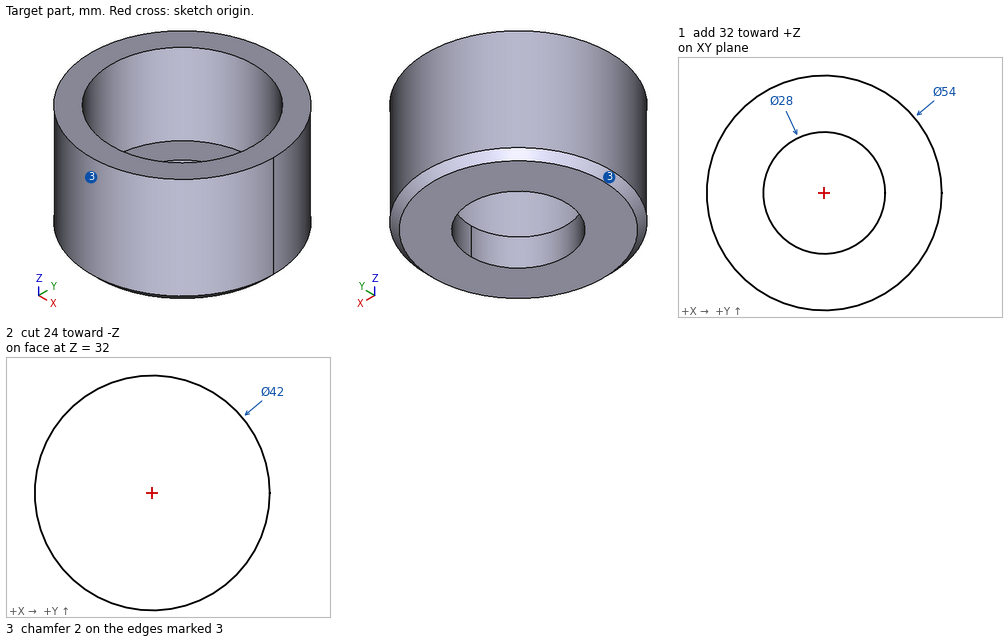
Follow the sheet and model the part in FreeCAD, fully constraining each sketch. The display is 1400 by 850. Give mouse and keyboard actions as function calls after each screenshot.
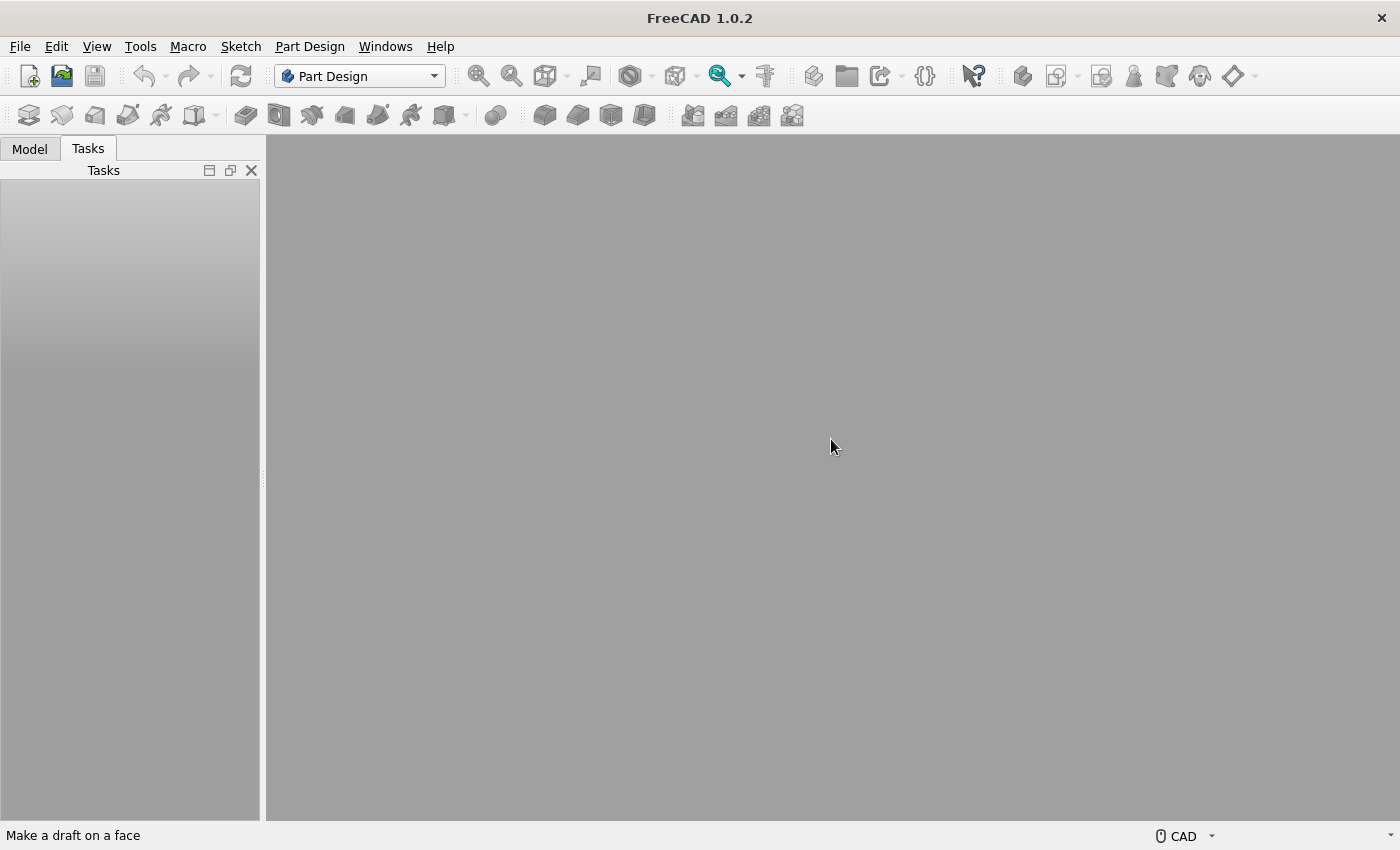
key(ctrl+n)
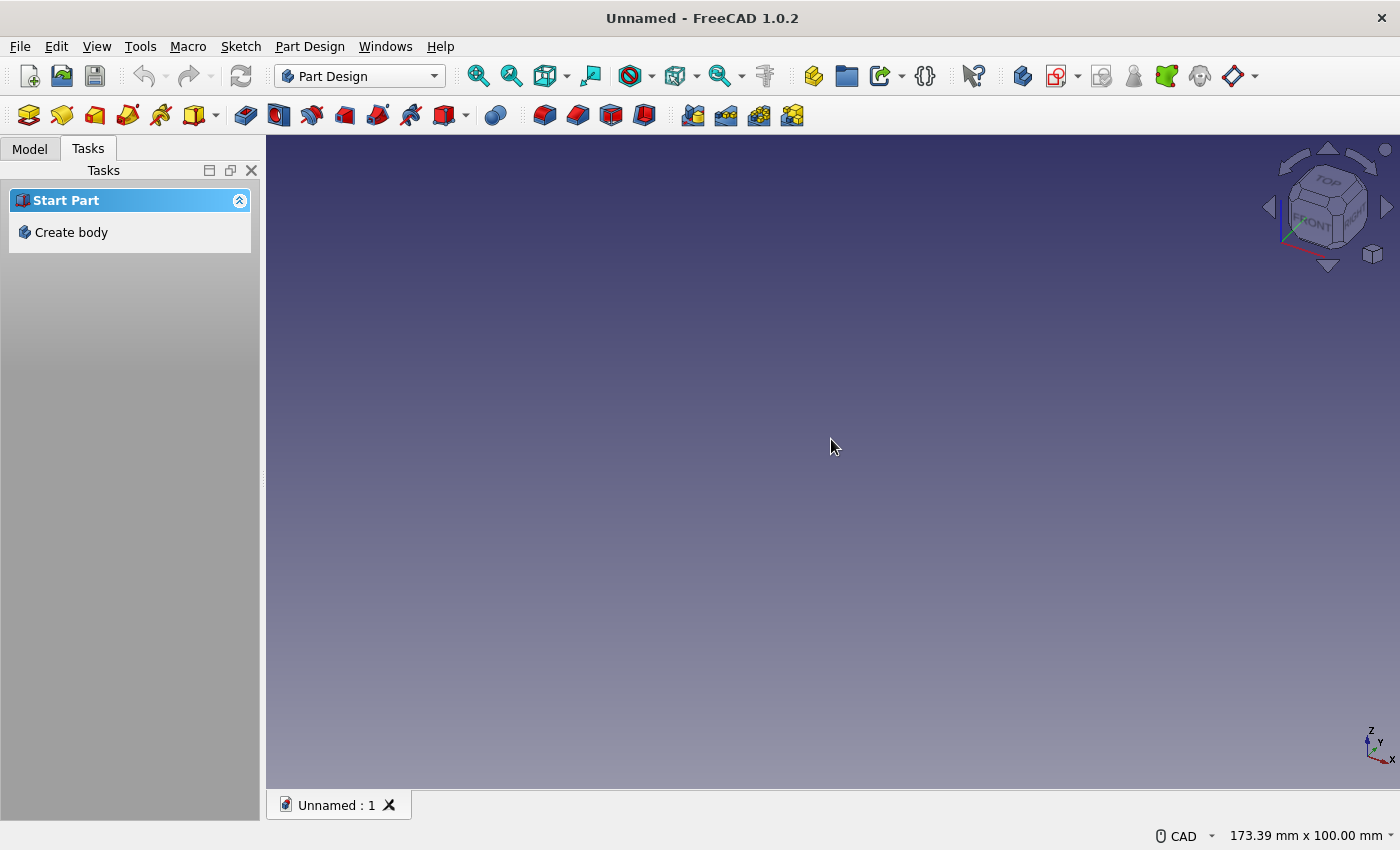
click(1056, 76)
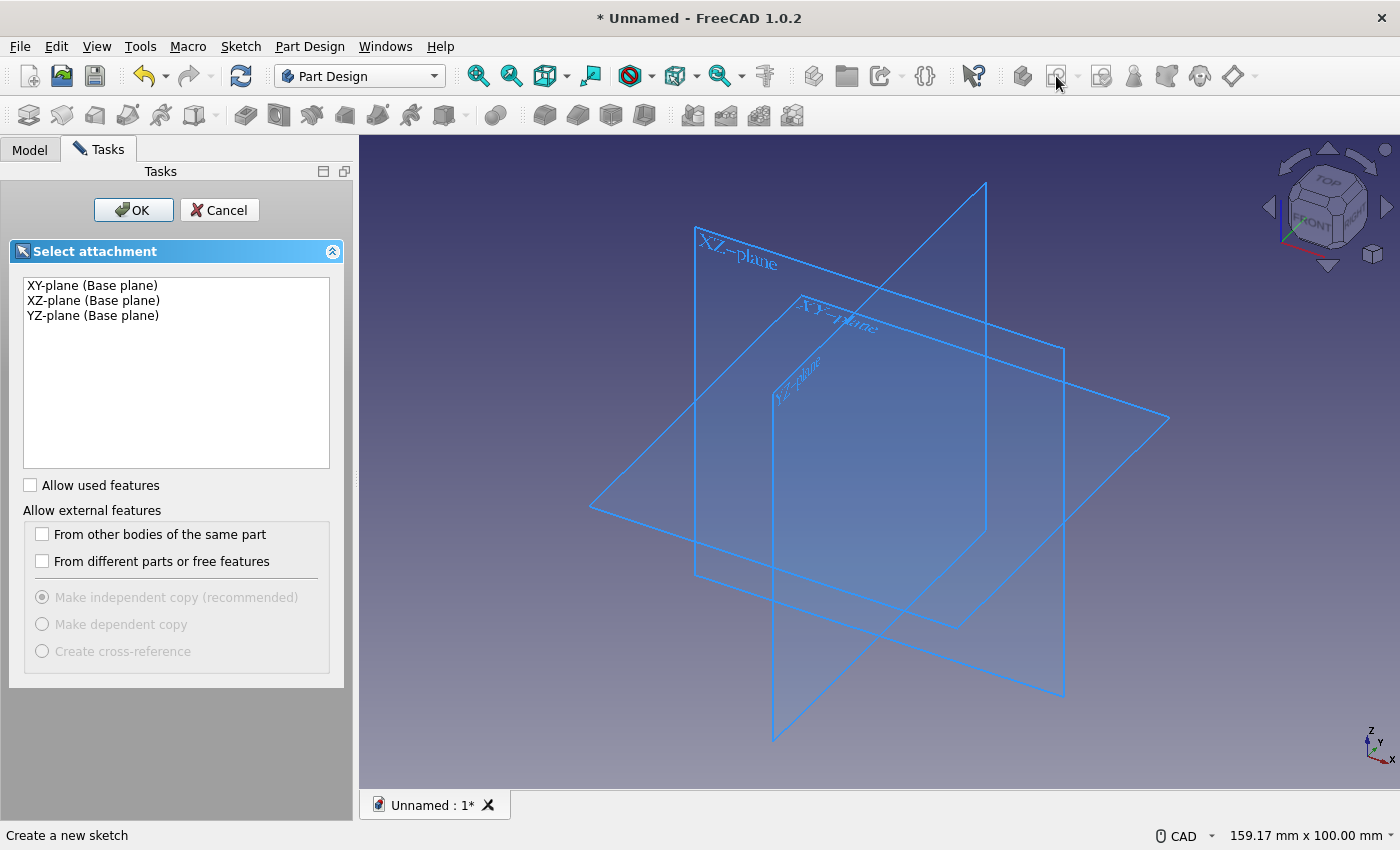
click(84, 286)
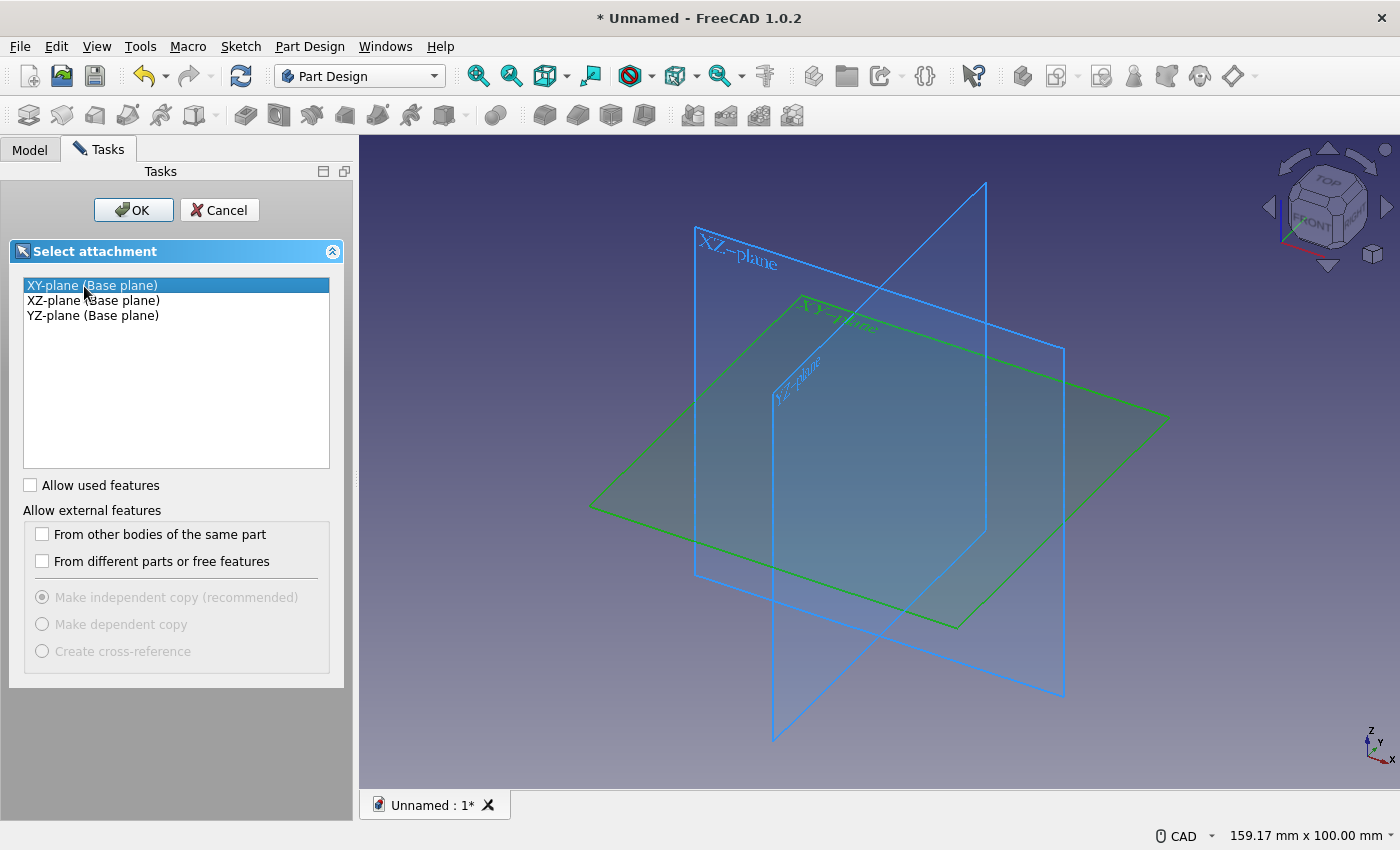
click(134, 210)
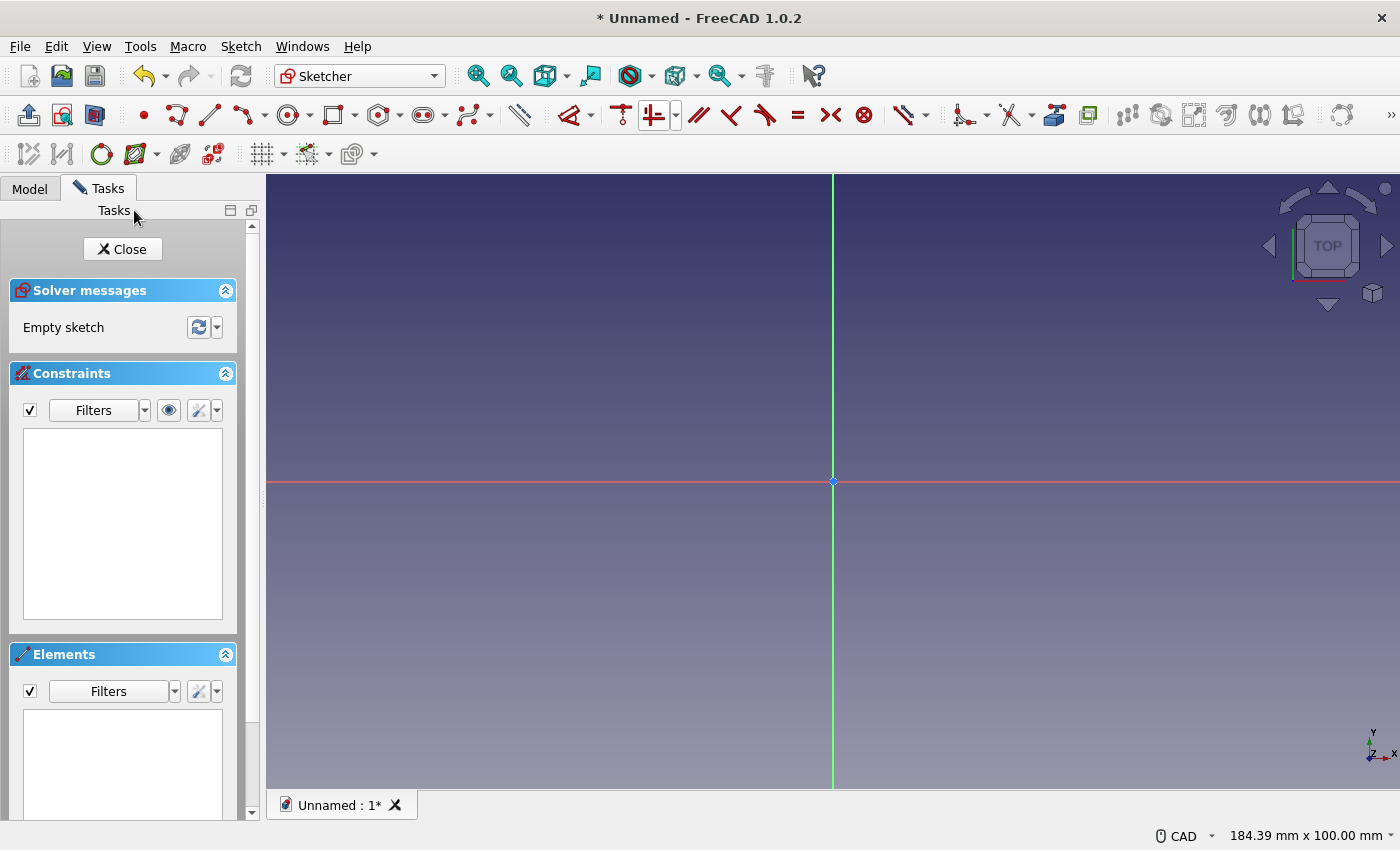
click(288, 116)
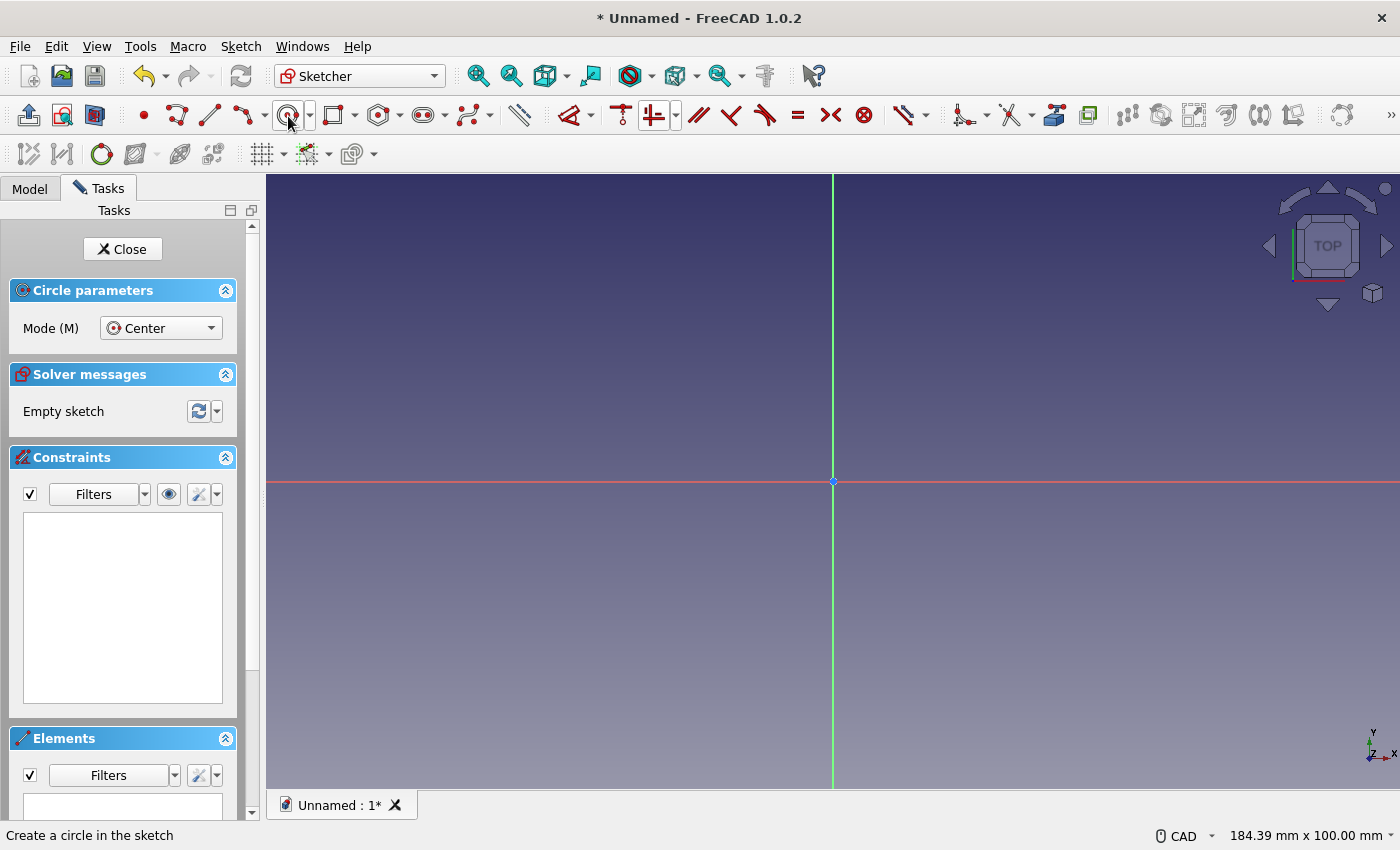
click(833, 482)
move(950, 364)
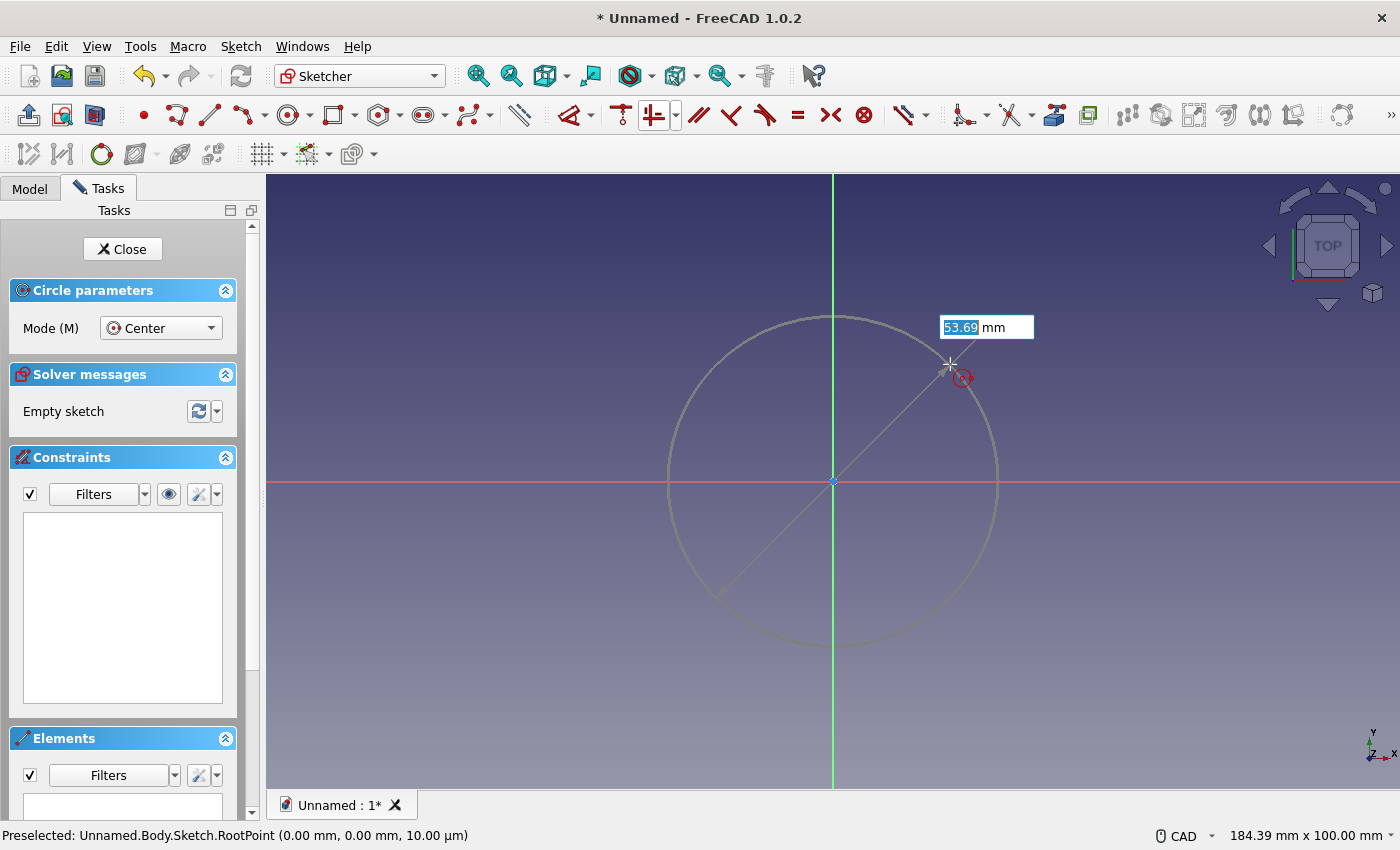
text(54)
key(Return)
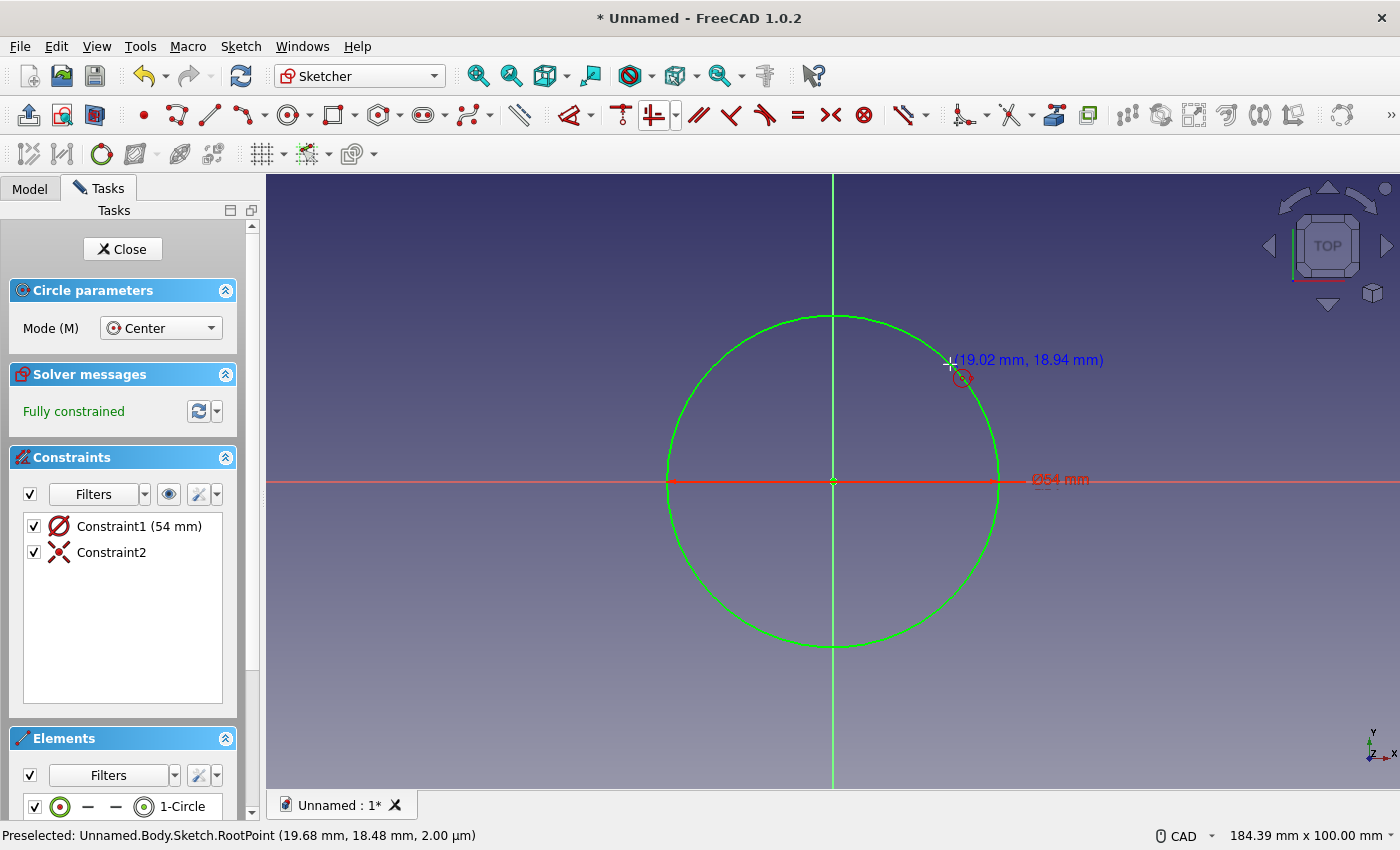
click(833, 482)
move(894, 421)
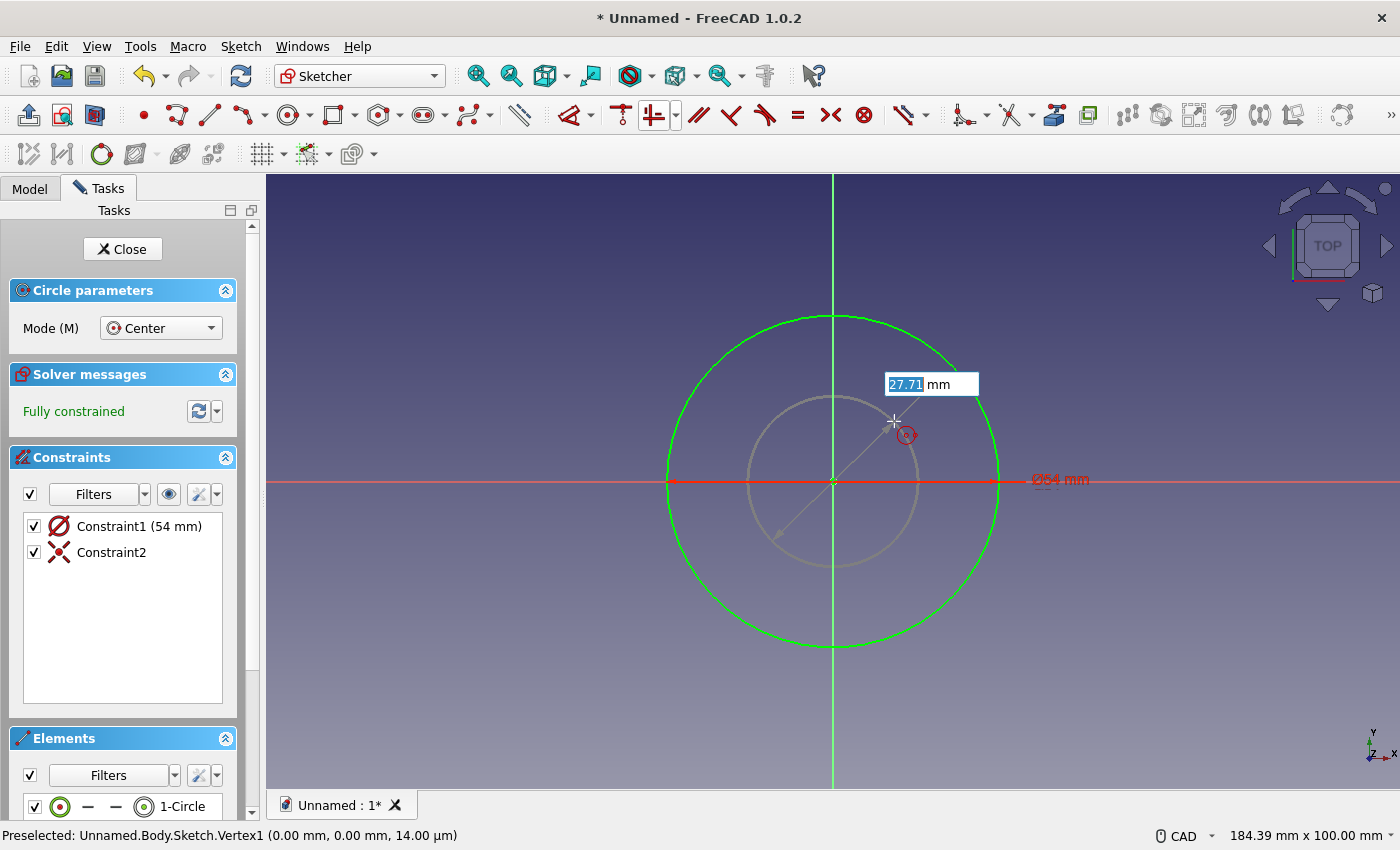
text(28)
key(Return)
key(Escape)